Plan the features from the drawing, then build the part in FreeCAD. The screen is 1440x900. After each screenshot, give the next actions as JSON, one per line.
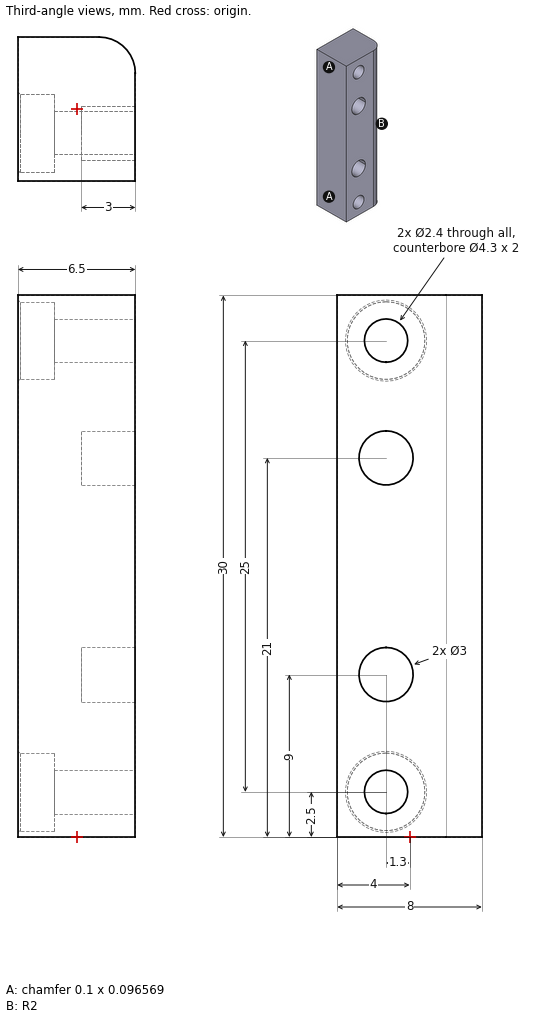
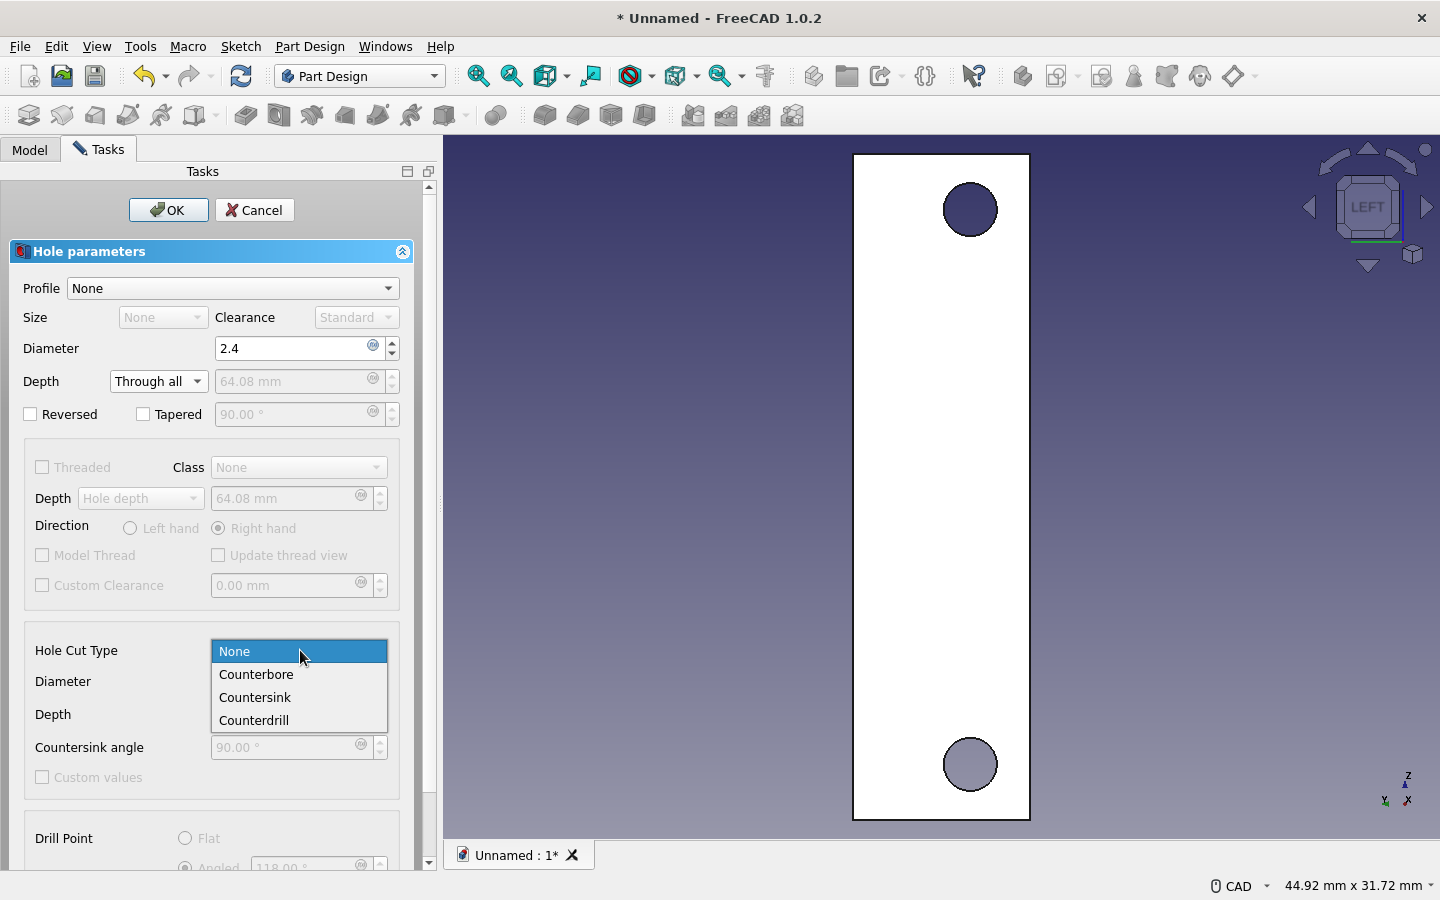
{"action": "left_click", "coordinate": [298, 674]}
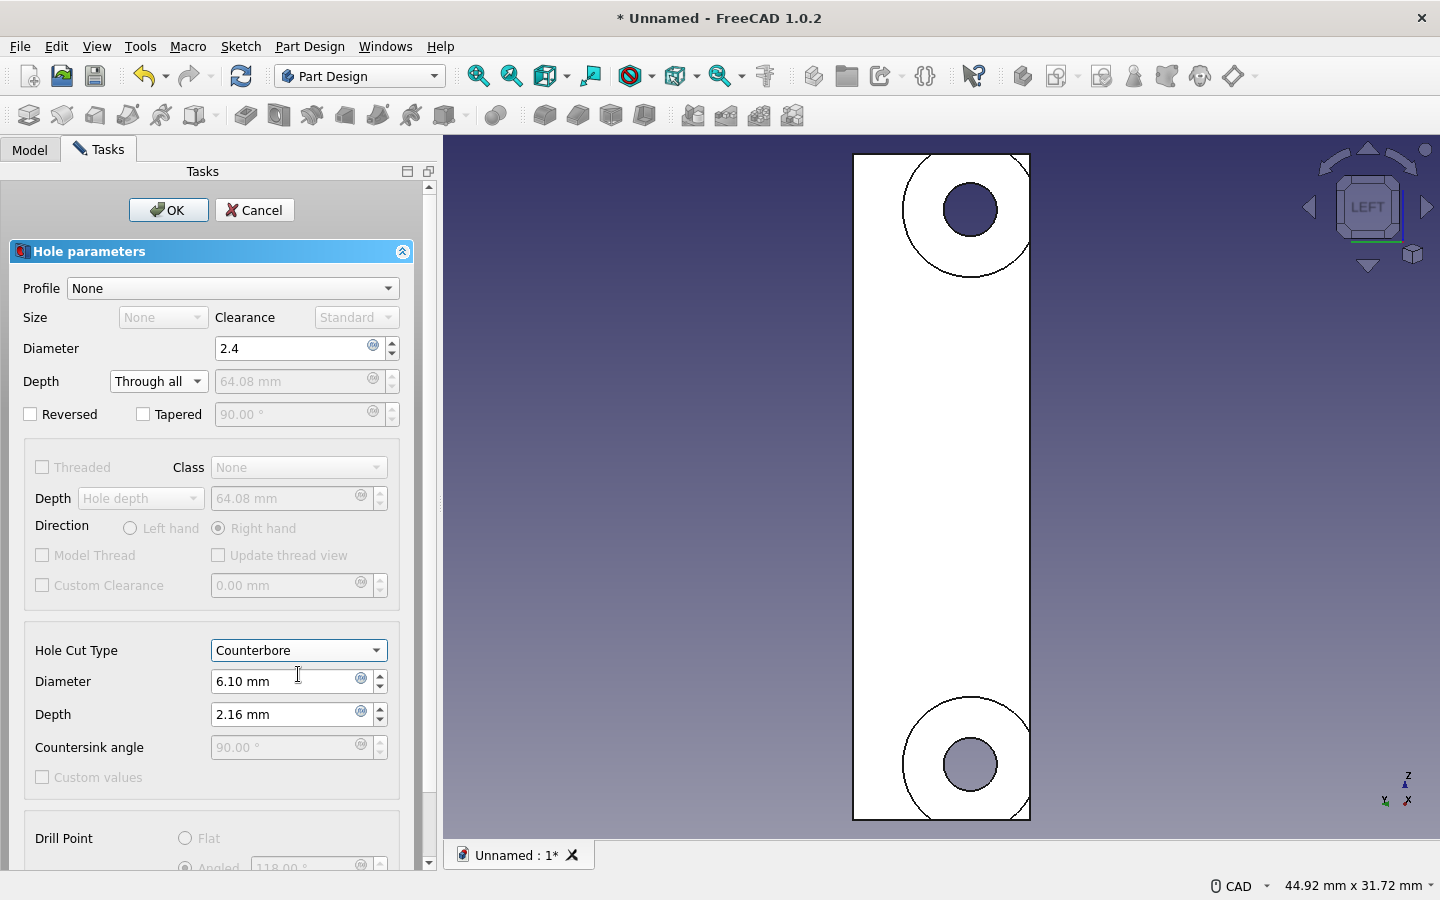
{"action": "triple_click", "coordinate": [292, 682]}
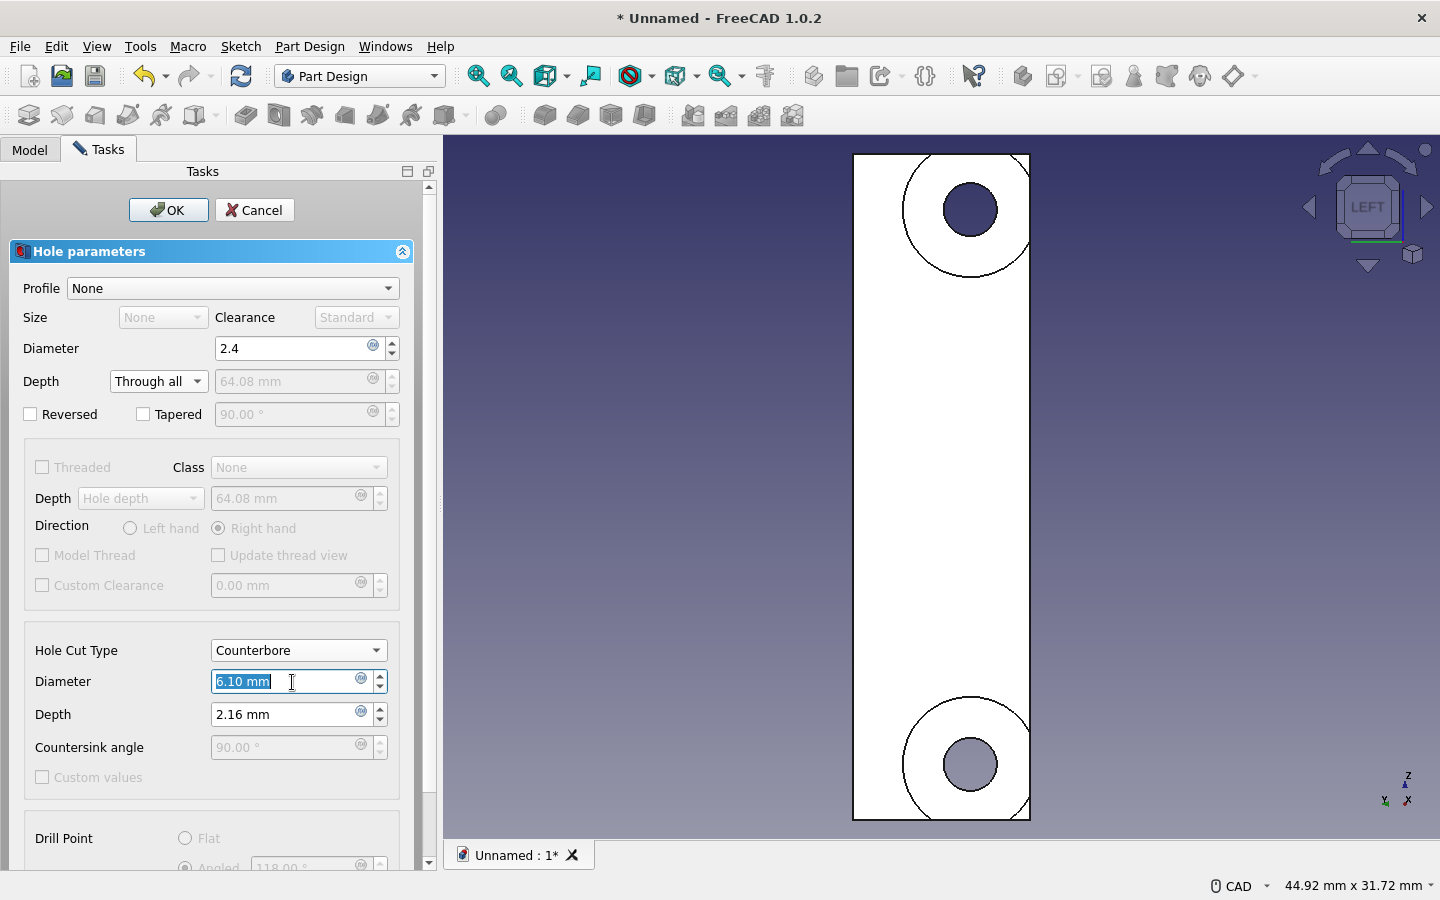
{"action": "type", "text": "4.3"}
{"action": "key", "text": "Tab"}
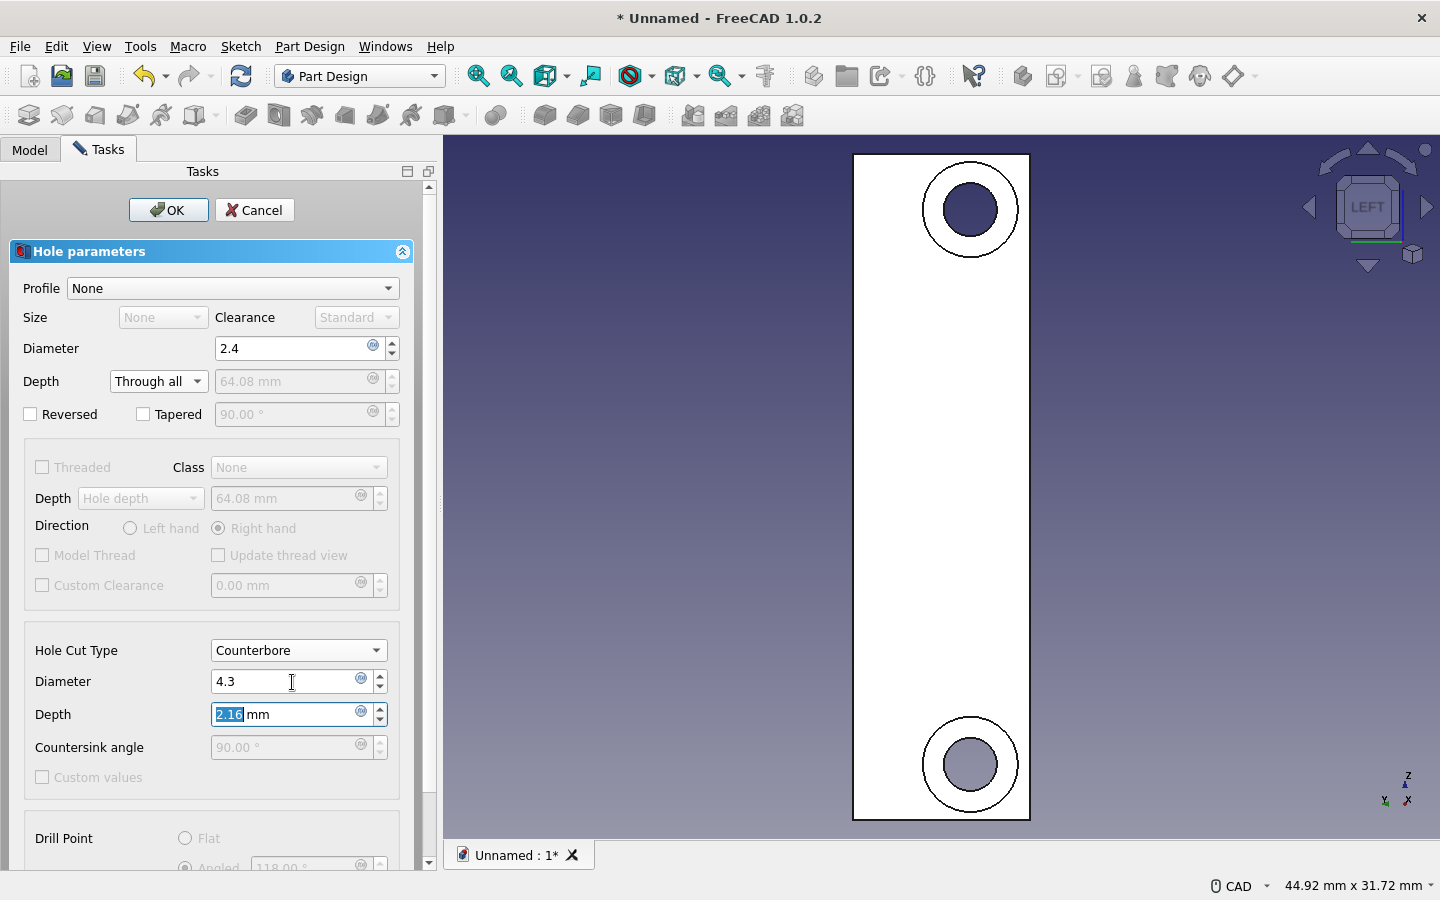
{"action": "type", "text": "2"}
{"action": "key", "text": "Tab"}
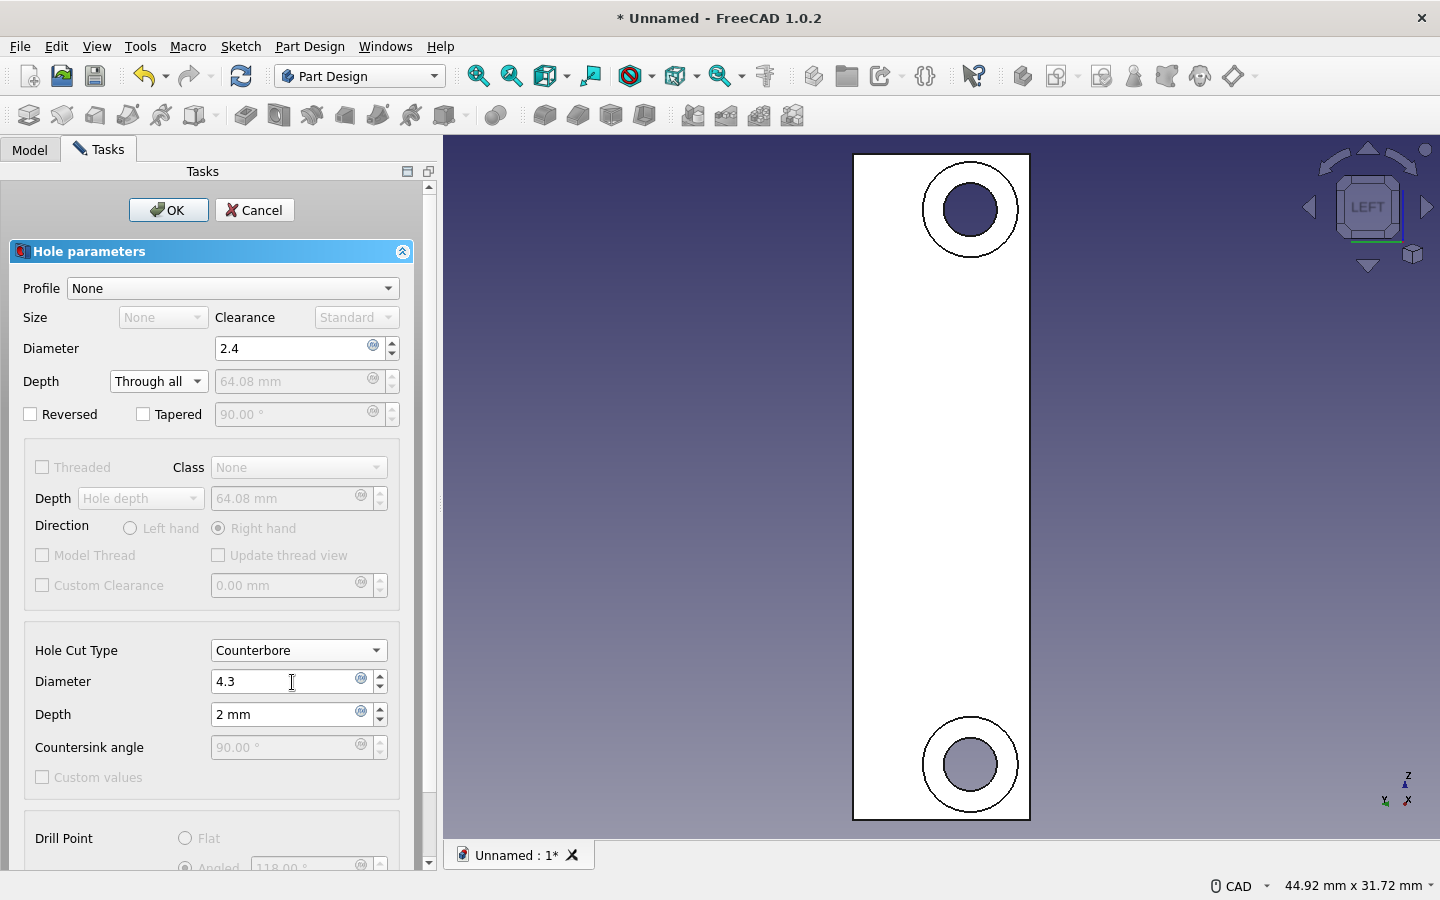
{"action": "left_click", "coordinate": [169, 210]}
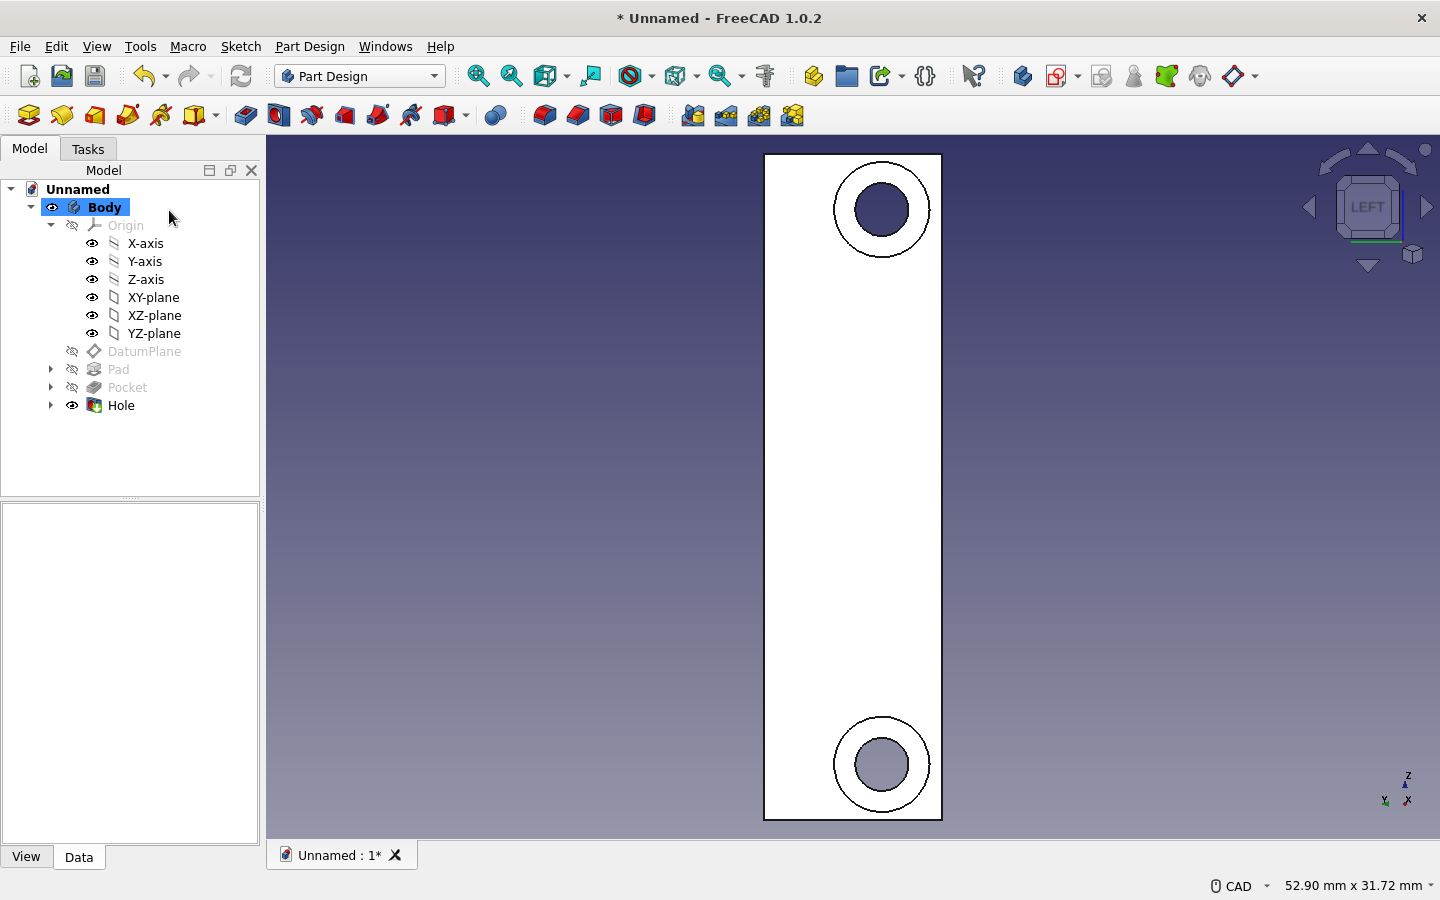
{"action": "left_click", "coordinate": [834, 763]}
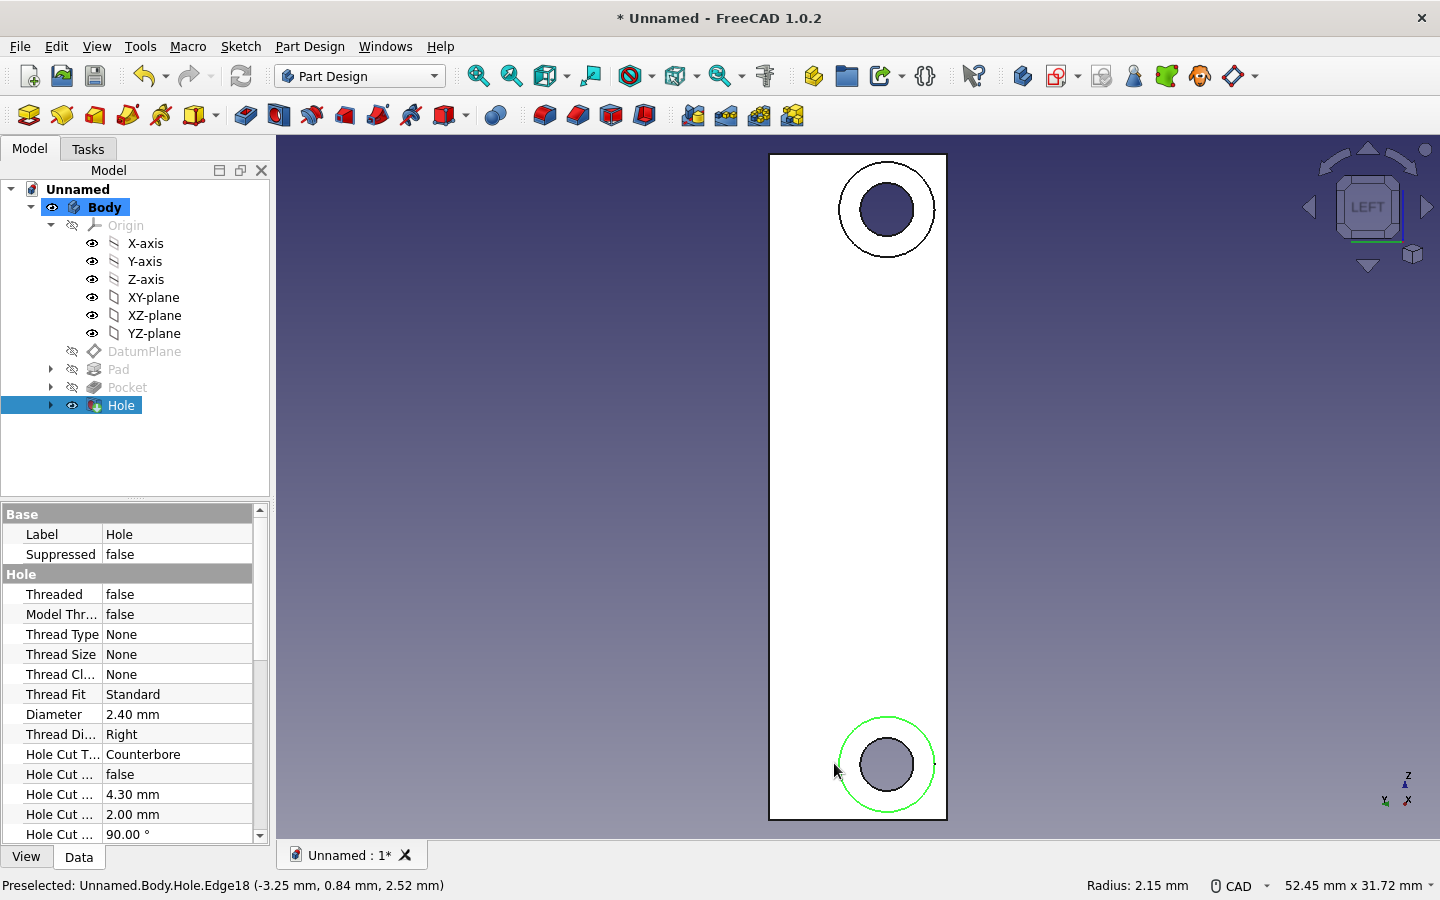
{"action": "left_click", "coordinate": [839, 209], "text": "ctrl"}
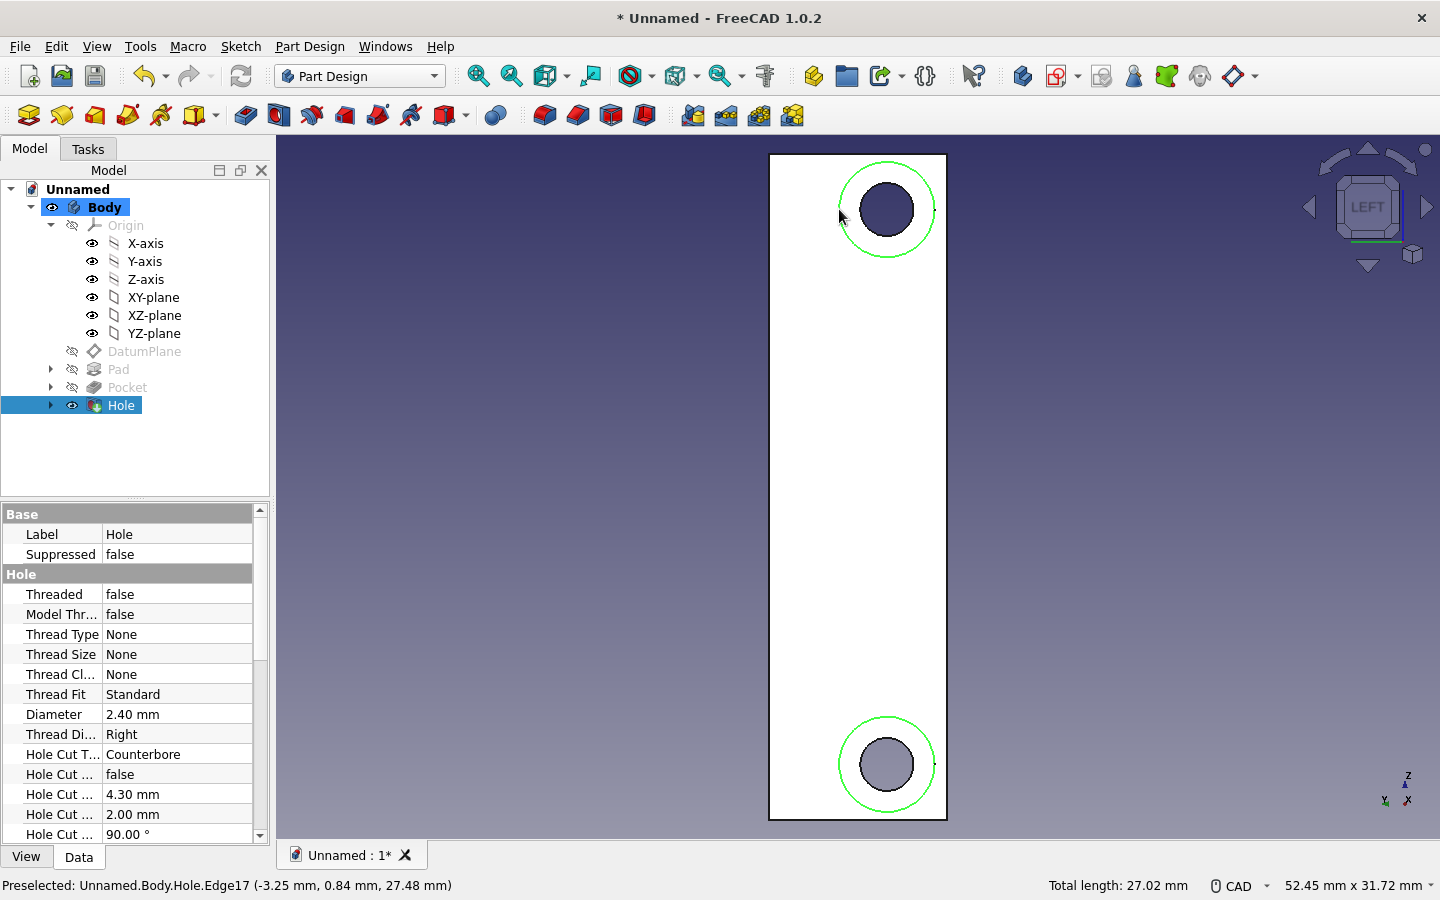
{"action": "left_click", "coordinate": [578, 116]}